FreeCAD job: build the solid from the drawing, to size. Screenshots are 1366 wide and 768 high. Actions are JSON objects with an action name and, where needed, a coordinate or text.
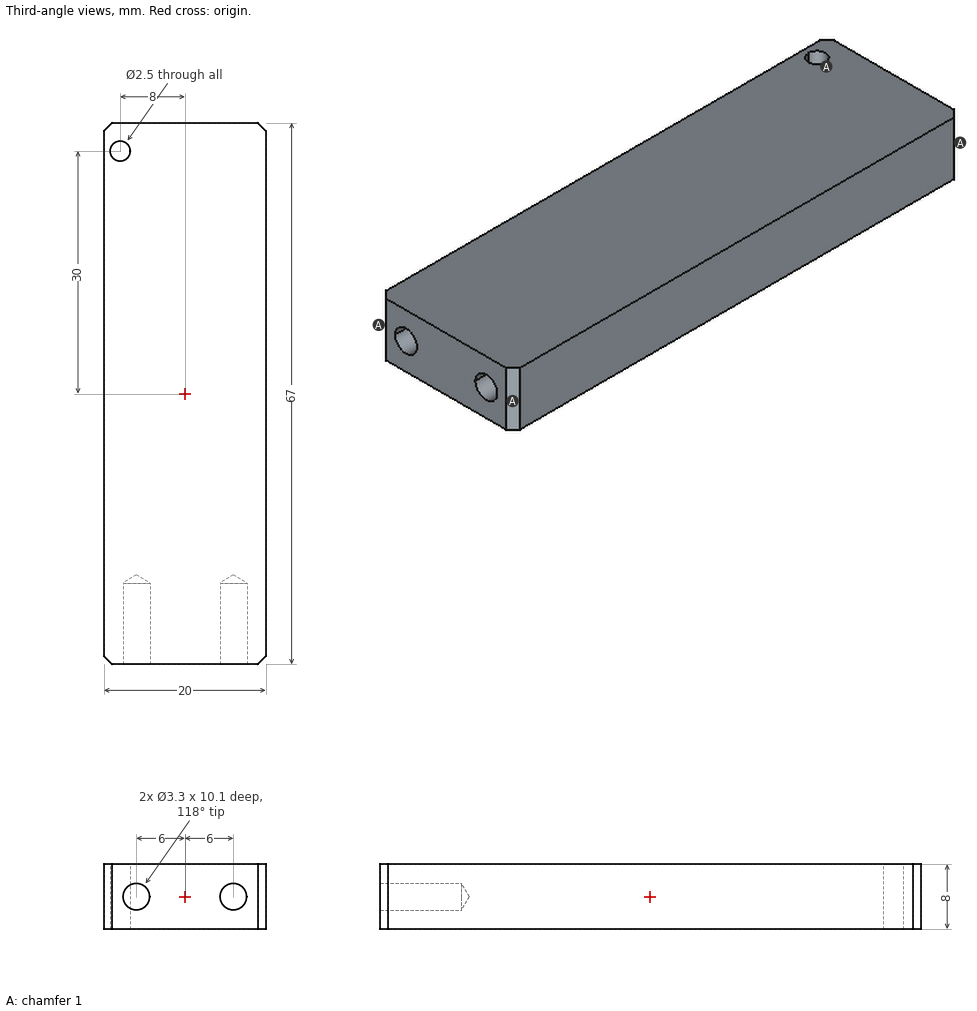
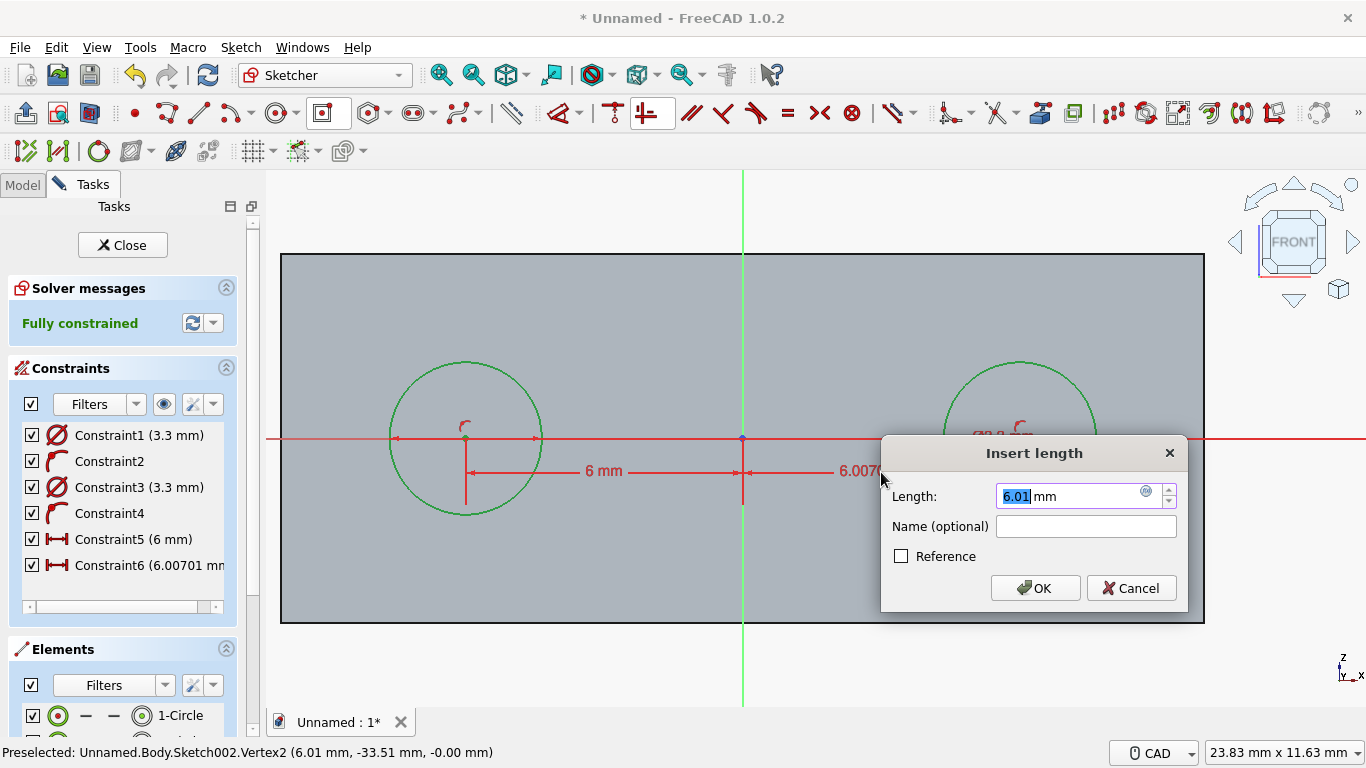
{"action": "type", "text": "6"}
{"action": "key", "text": "Return"}
{"action": "key", "text": "Escape"}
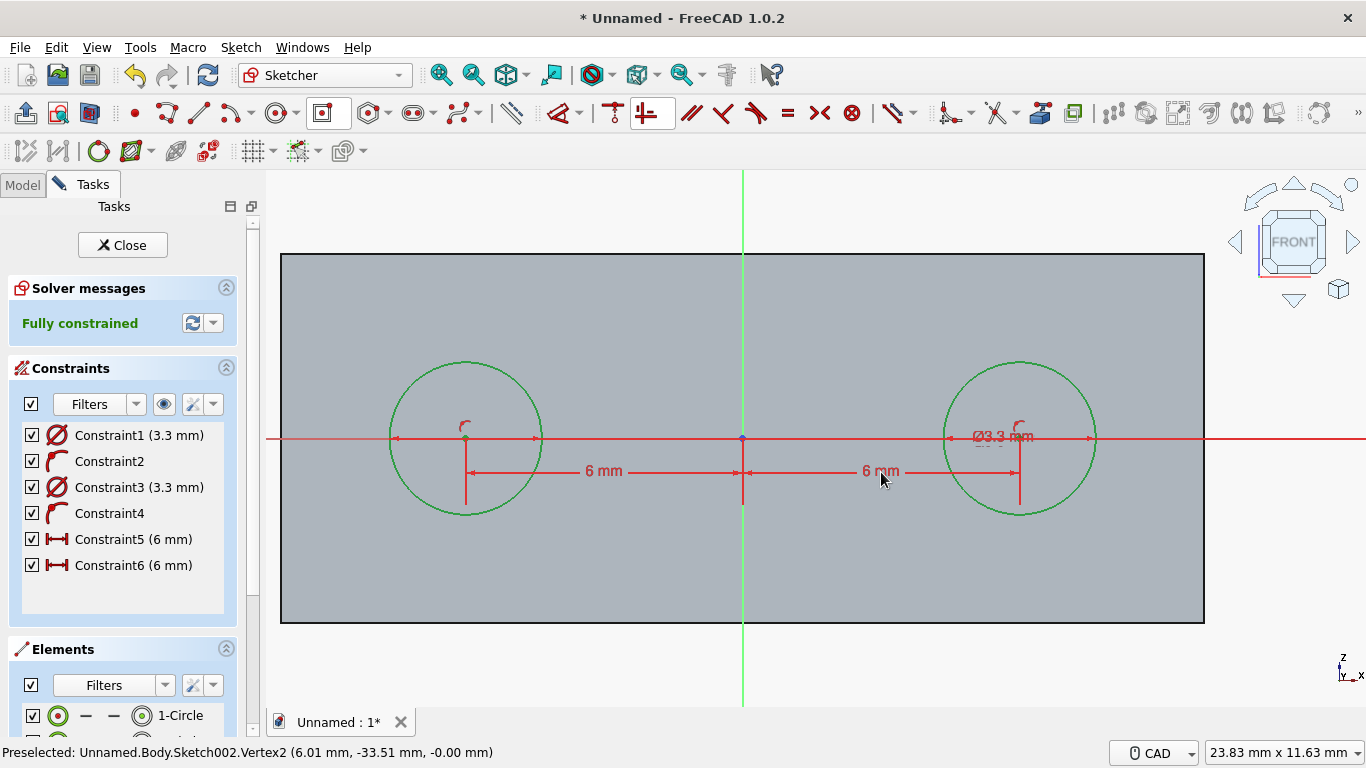
{"action": "left_click", "coordinate": [123, 245]}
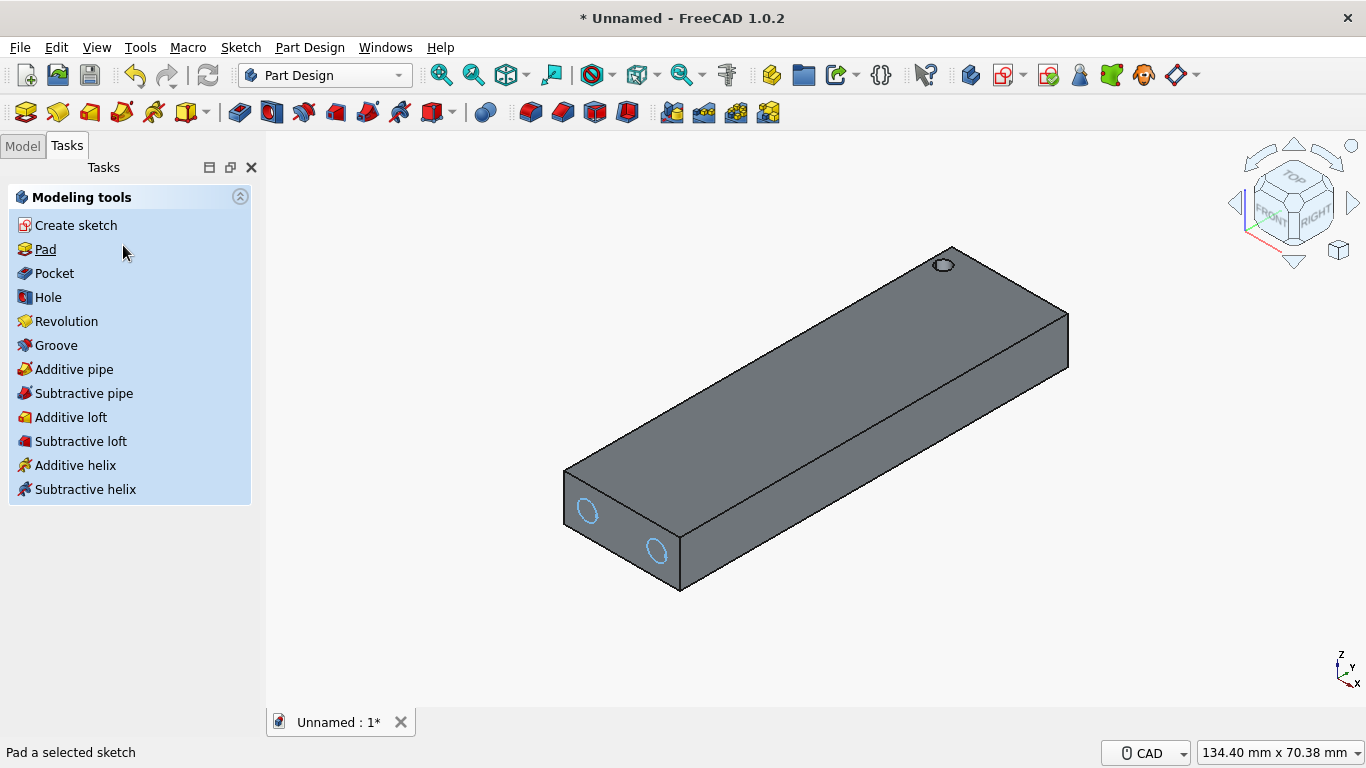
{"action": "left_click", "coordinate": [272, 112]}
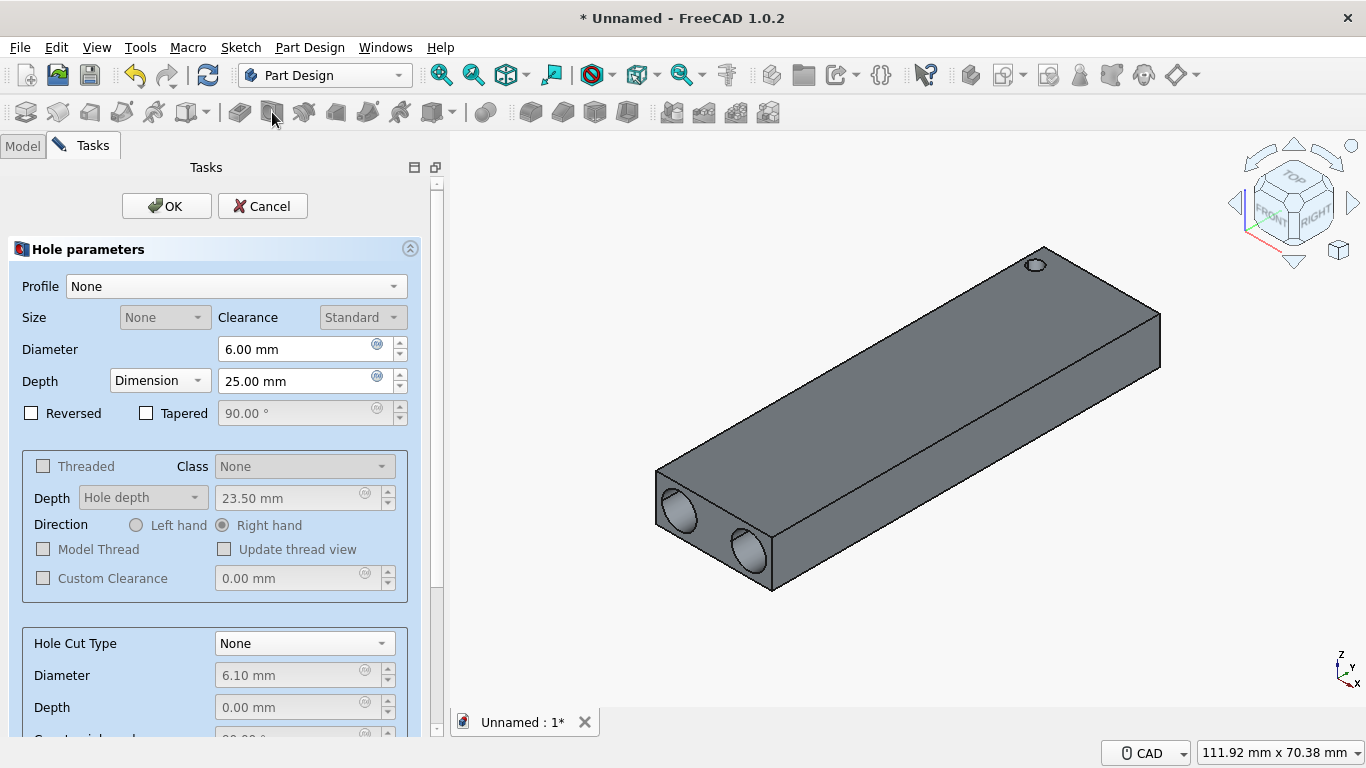
{"action": "triple_click", "coordinate": [305, 349]}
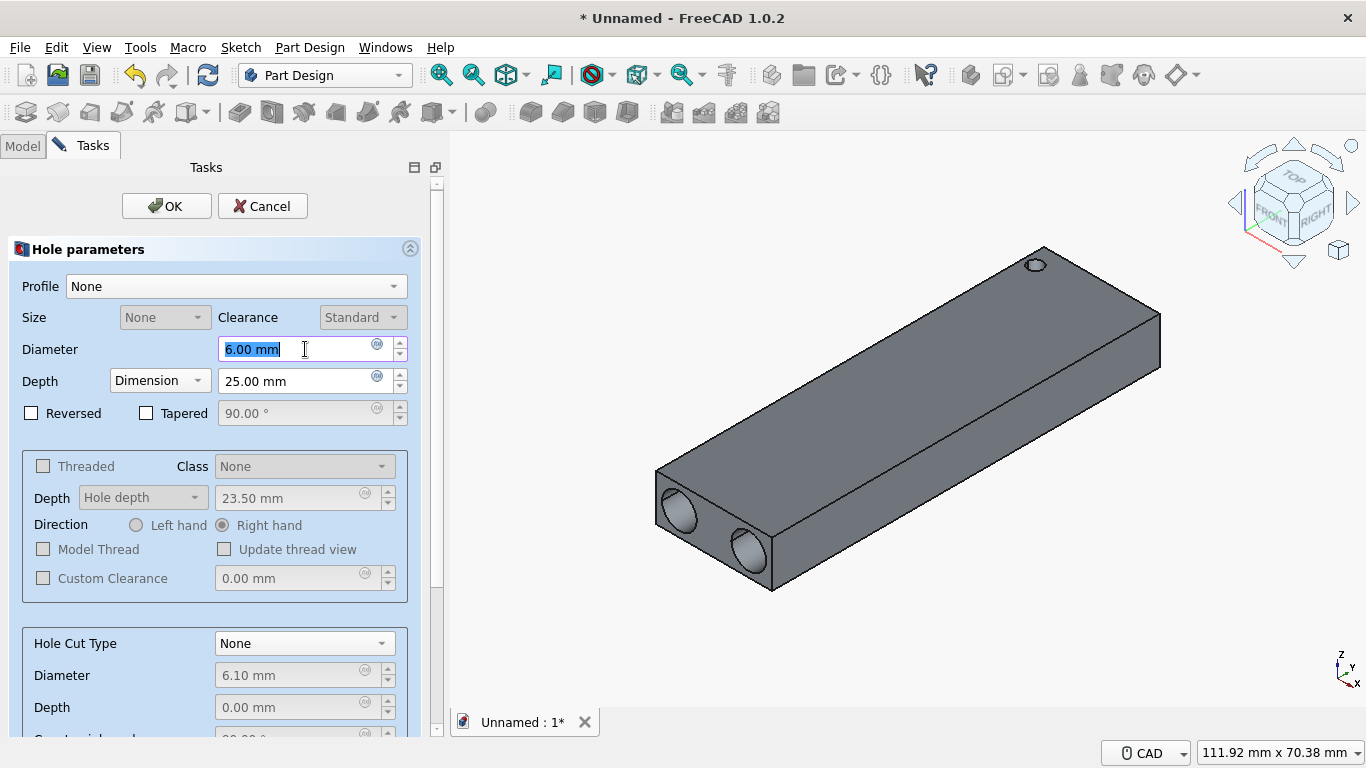
{"action": "type", "text": "3.3"}
{"action": "key", "text": "Tab"}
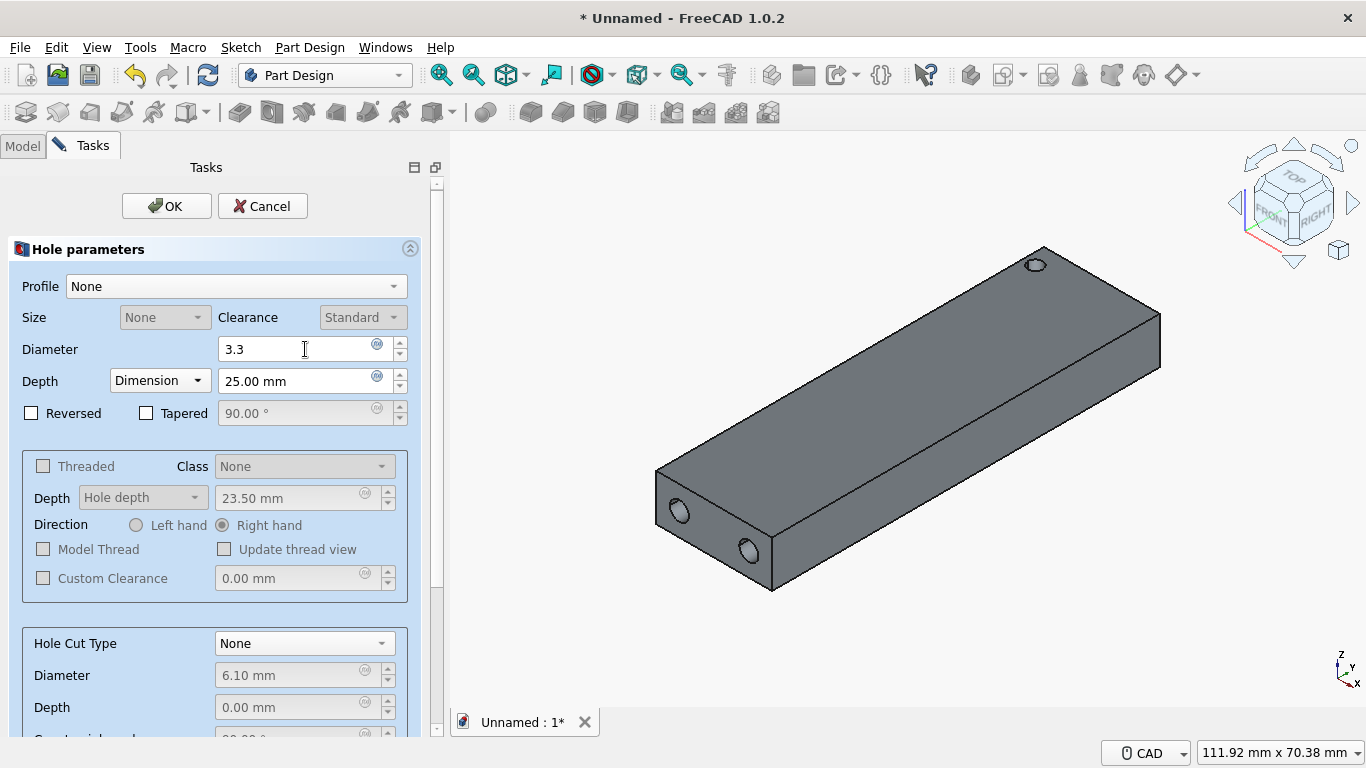
{"action": "triple_click", "coordinate": [305, 381]}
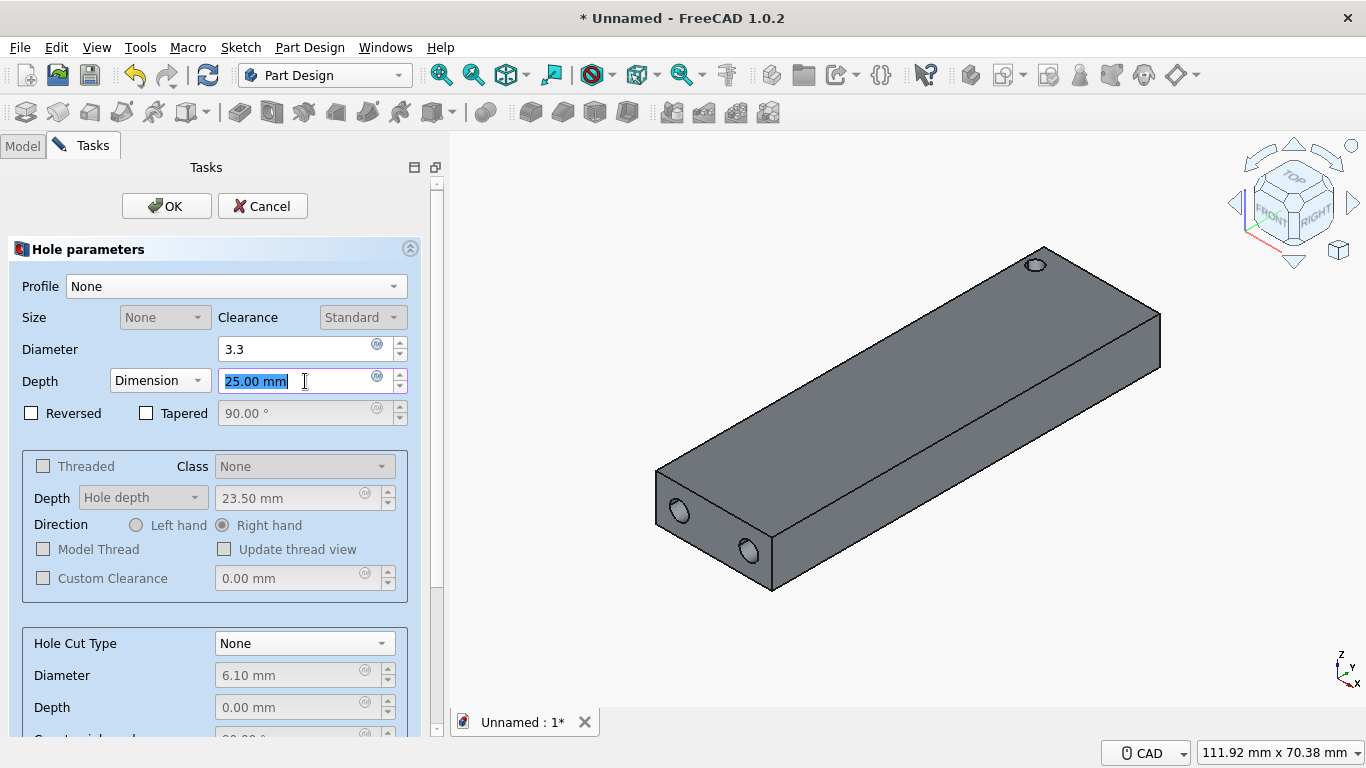
{"action": "type", "text": "10.1"}
{"action": "key", "text": "Tab"}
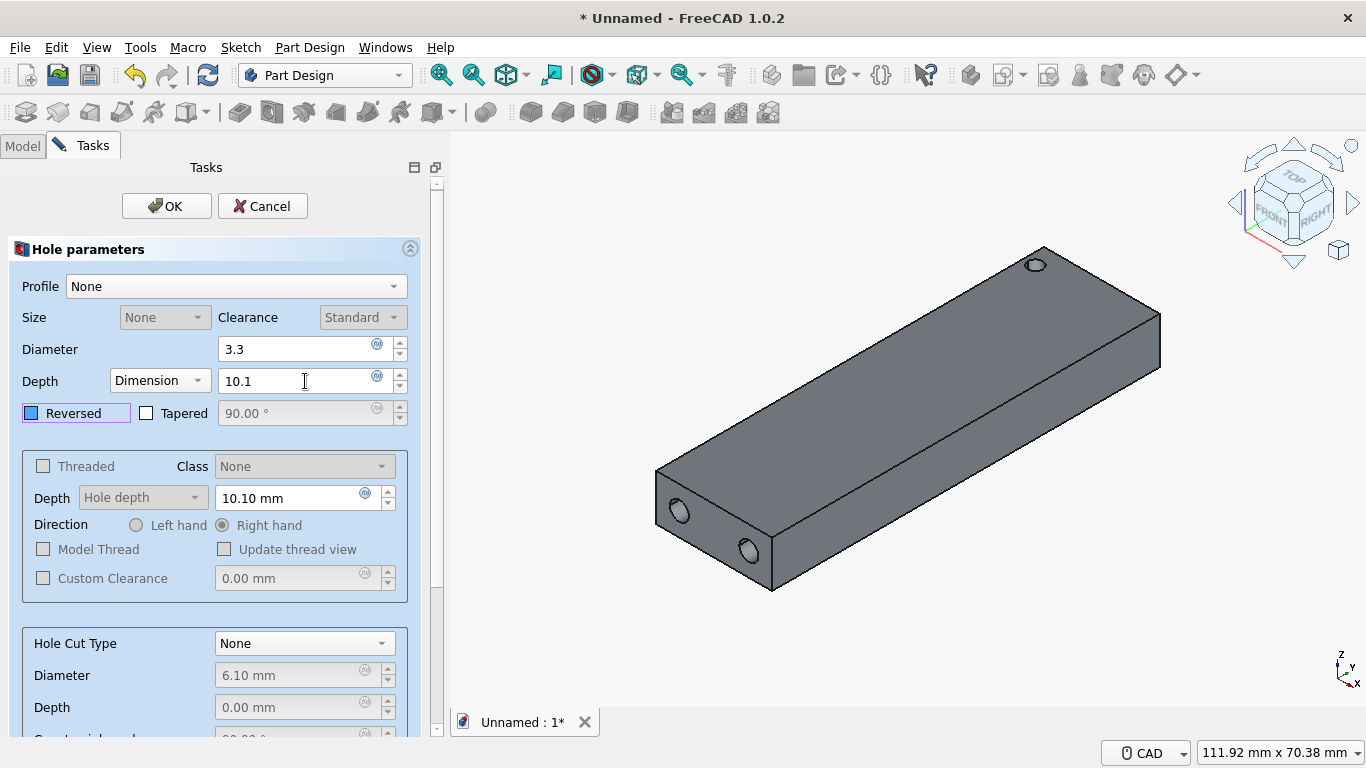
{"action": "left_click", "coordinate": [167, 206]}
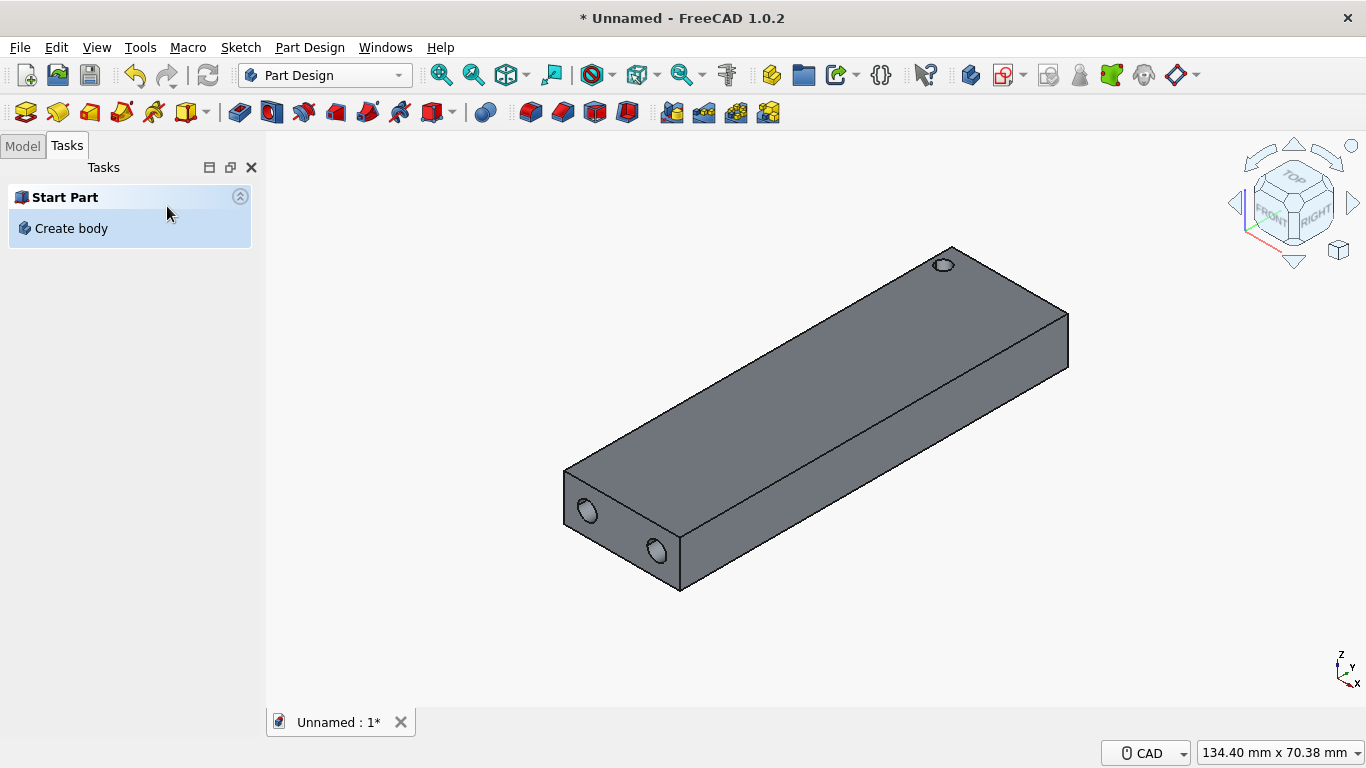
{"action": "left_click", "coordinate": [680, 563]}